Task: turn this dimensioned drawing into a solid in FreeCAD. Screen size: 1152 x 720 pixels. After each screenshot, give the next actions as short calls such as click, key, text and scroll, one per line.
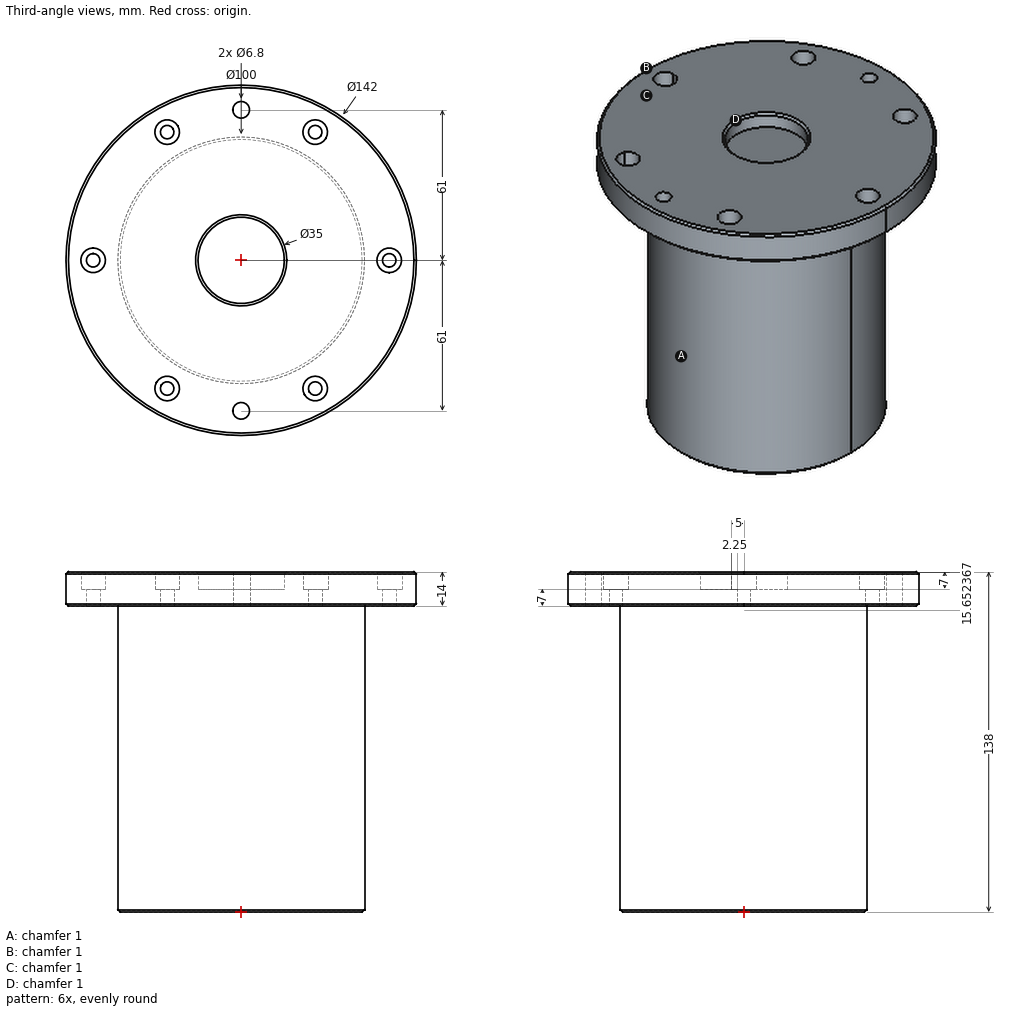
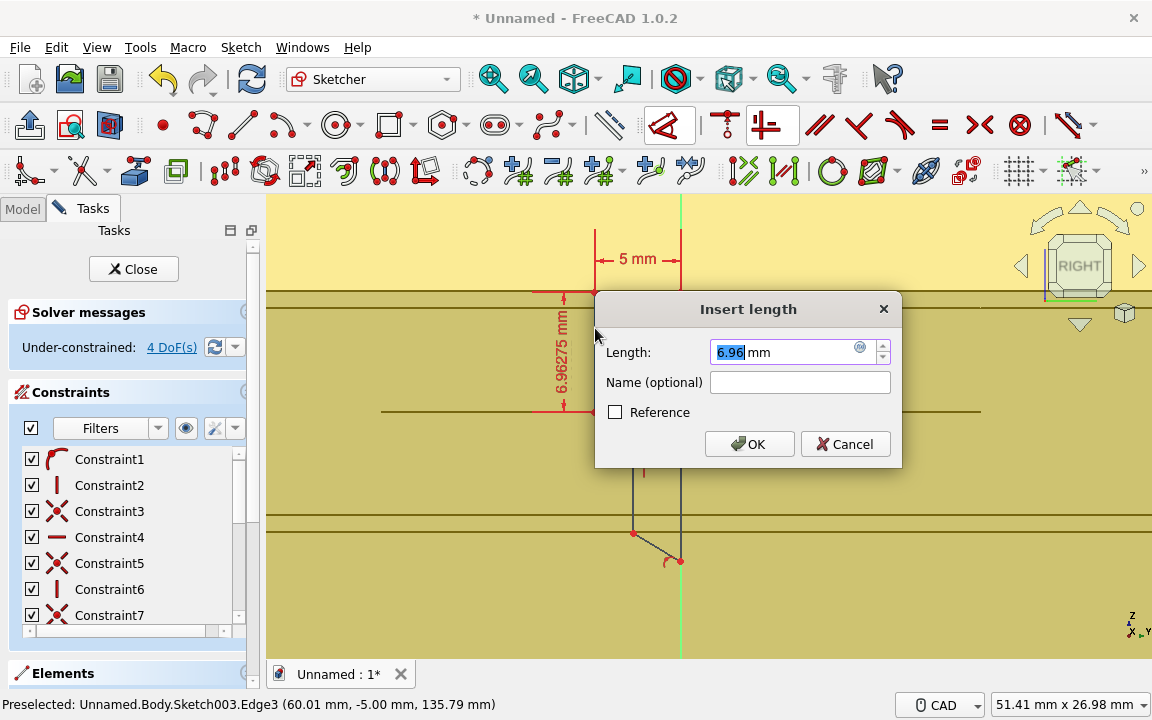
text(7)
key(Return)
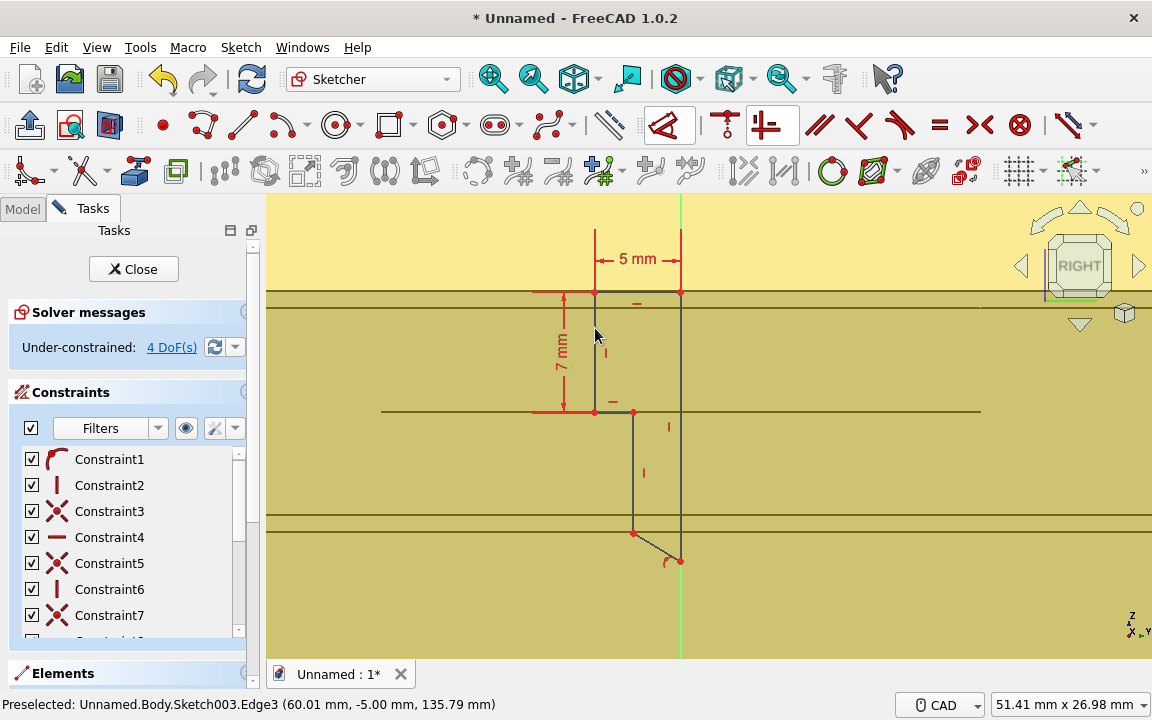
click(633, 449)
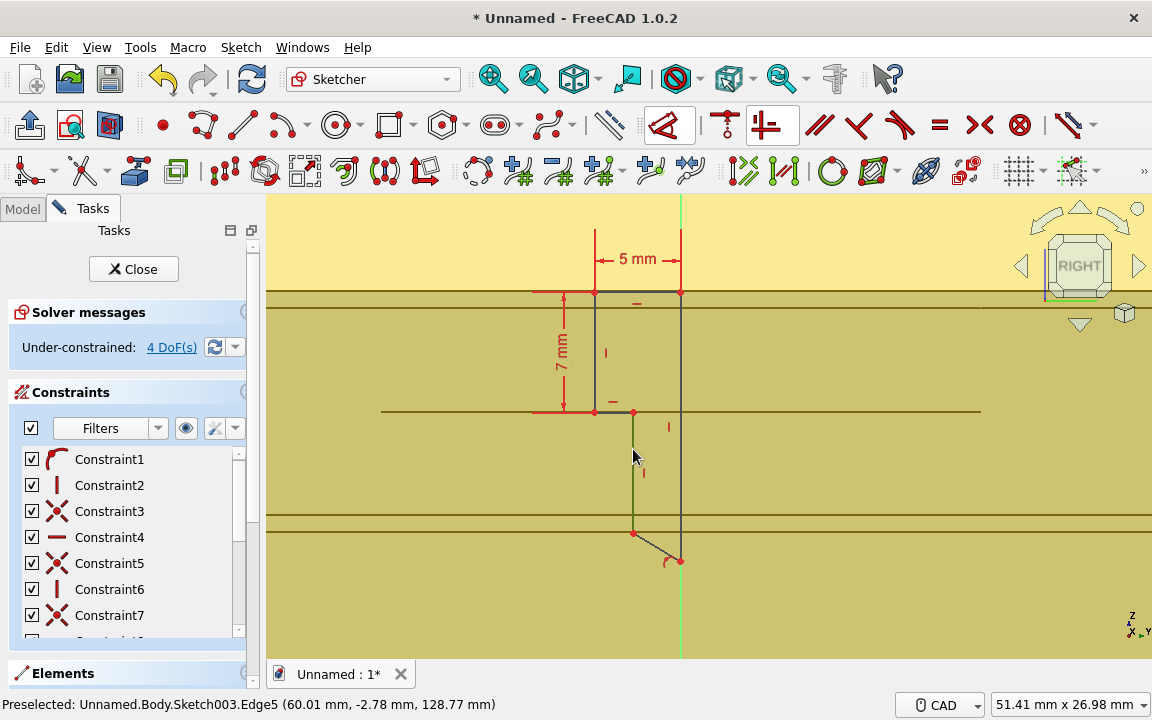
click(690, 126)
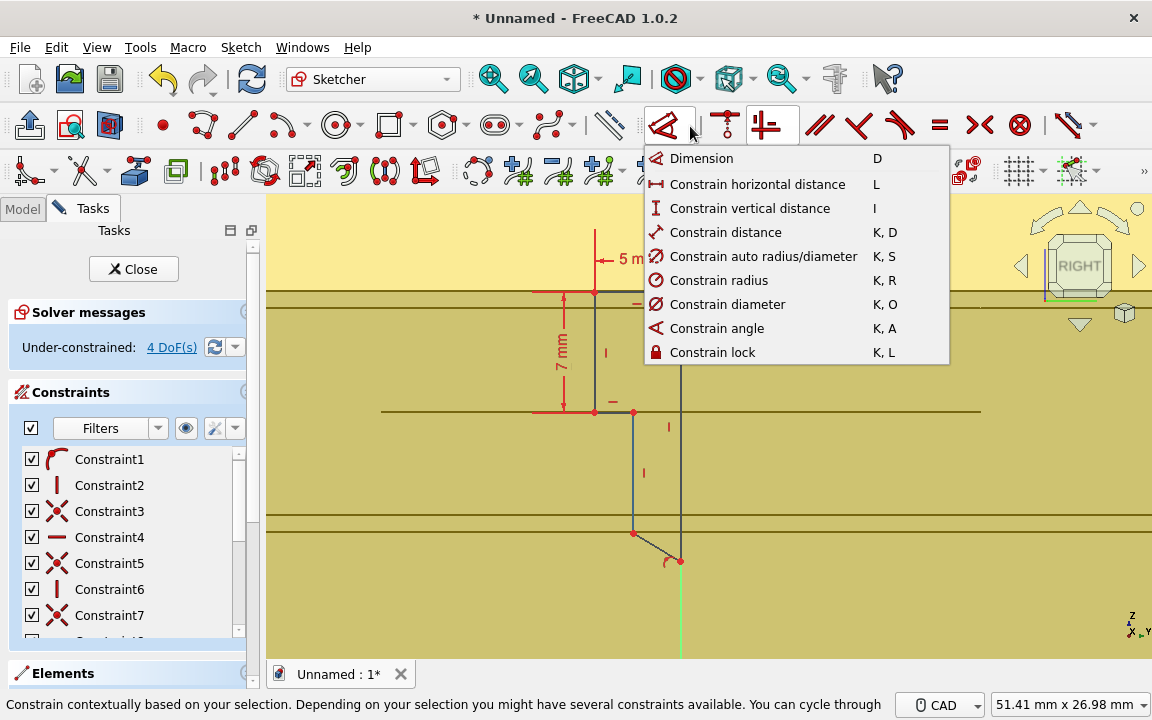
click(797, 208)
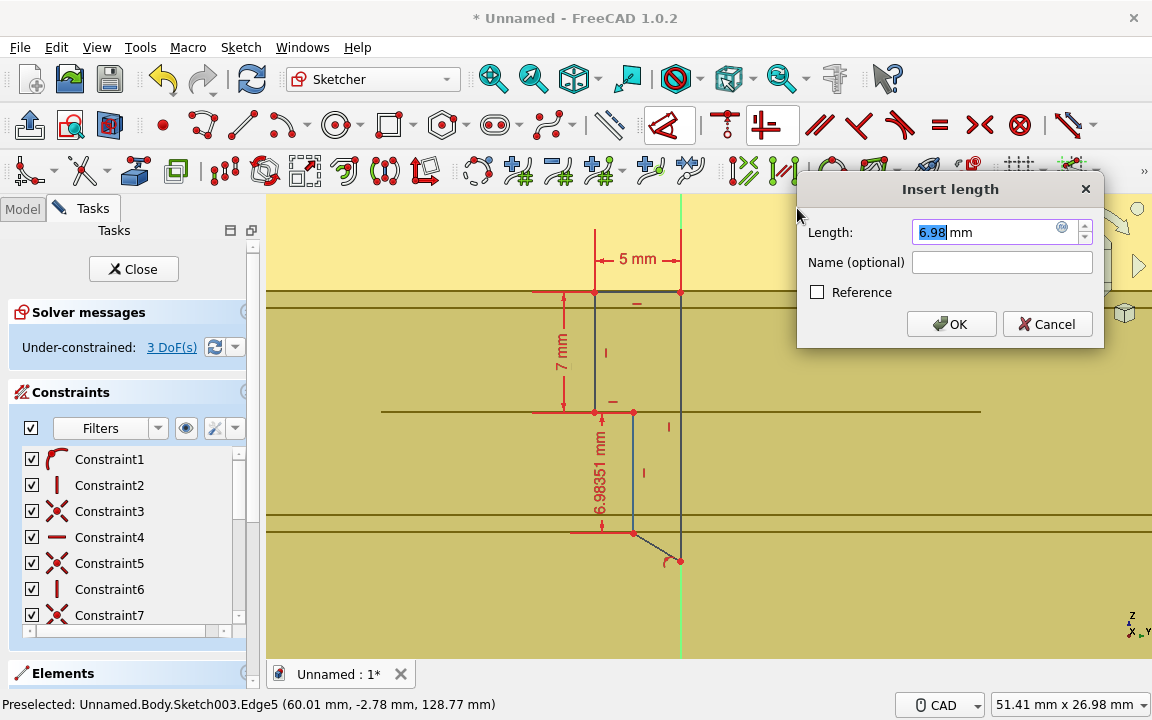
text(7)
key(Return)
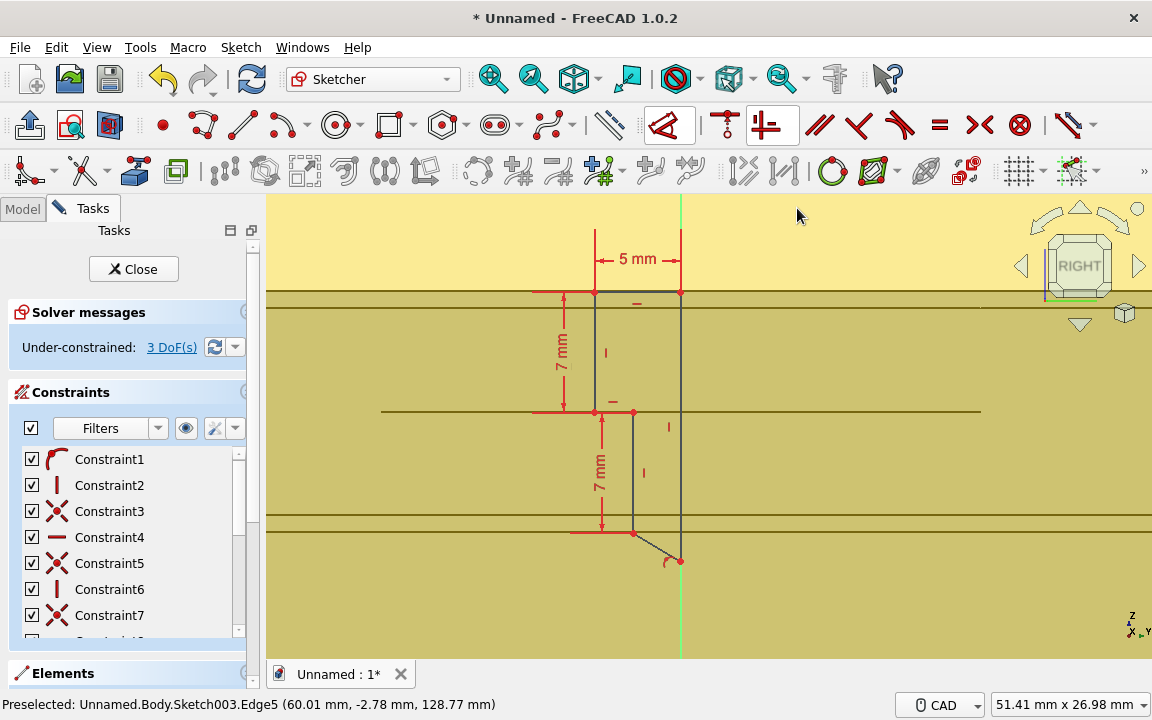
click(606, 413)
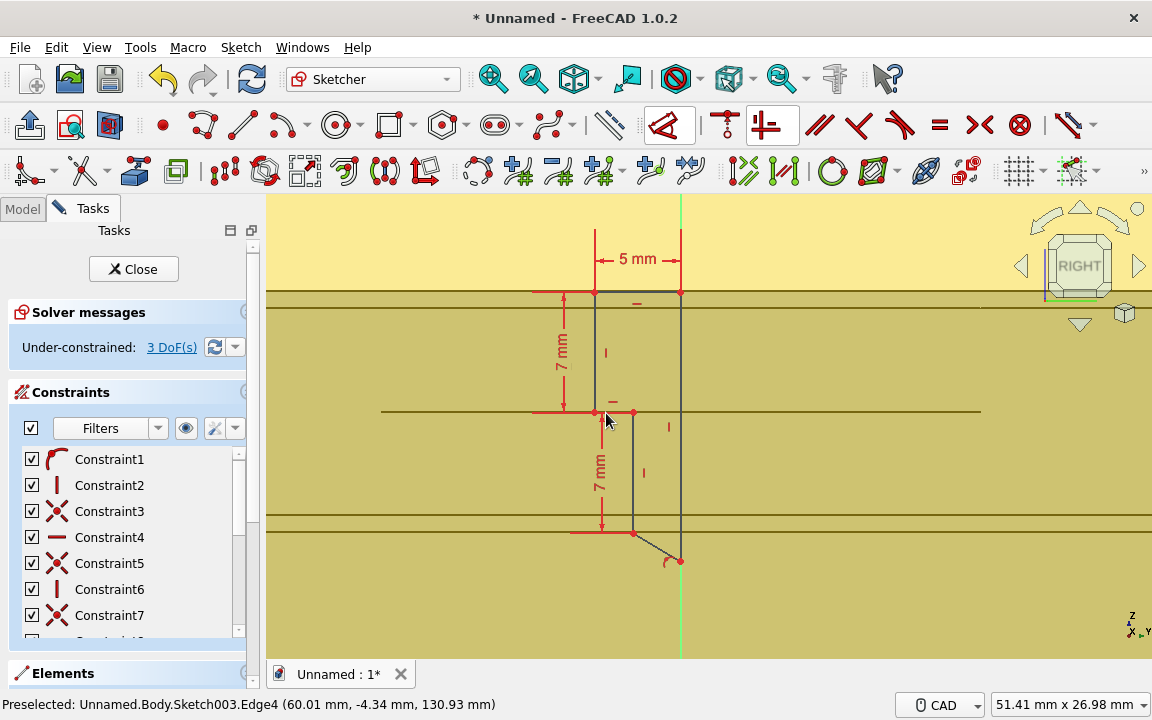
key(l)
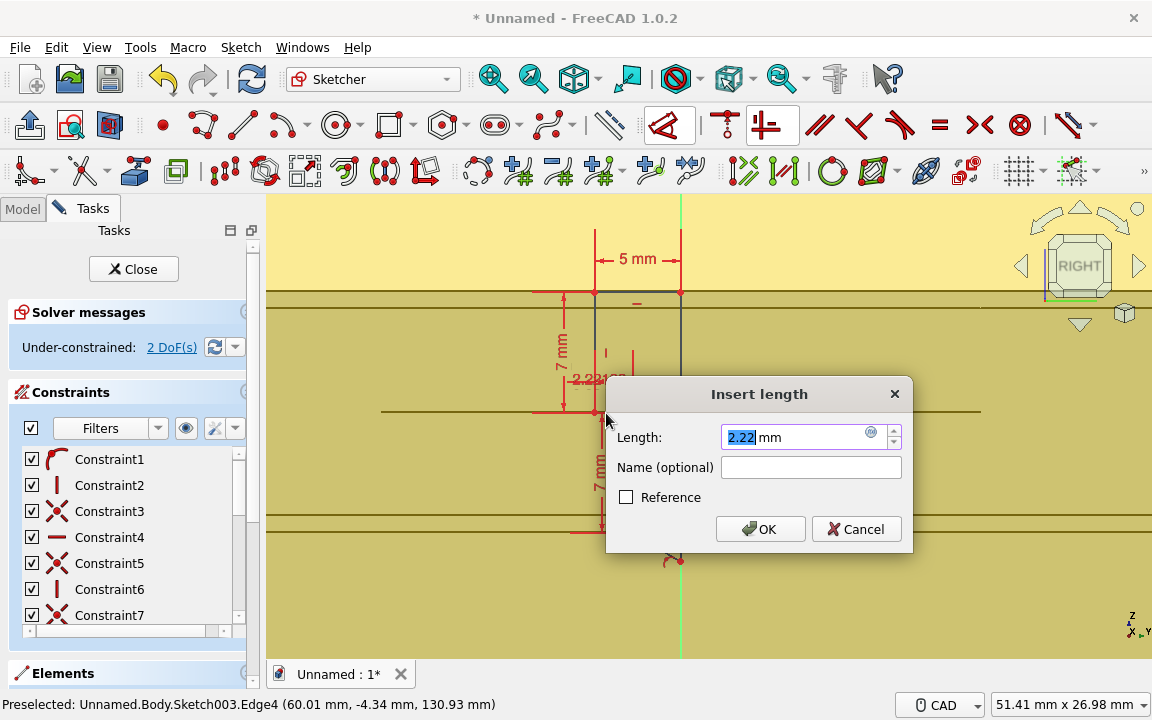
text(2.25)
key(Return)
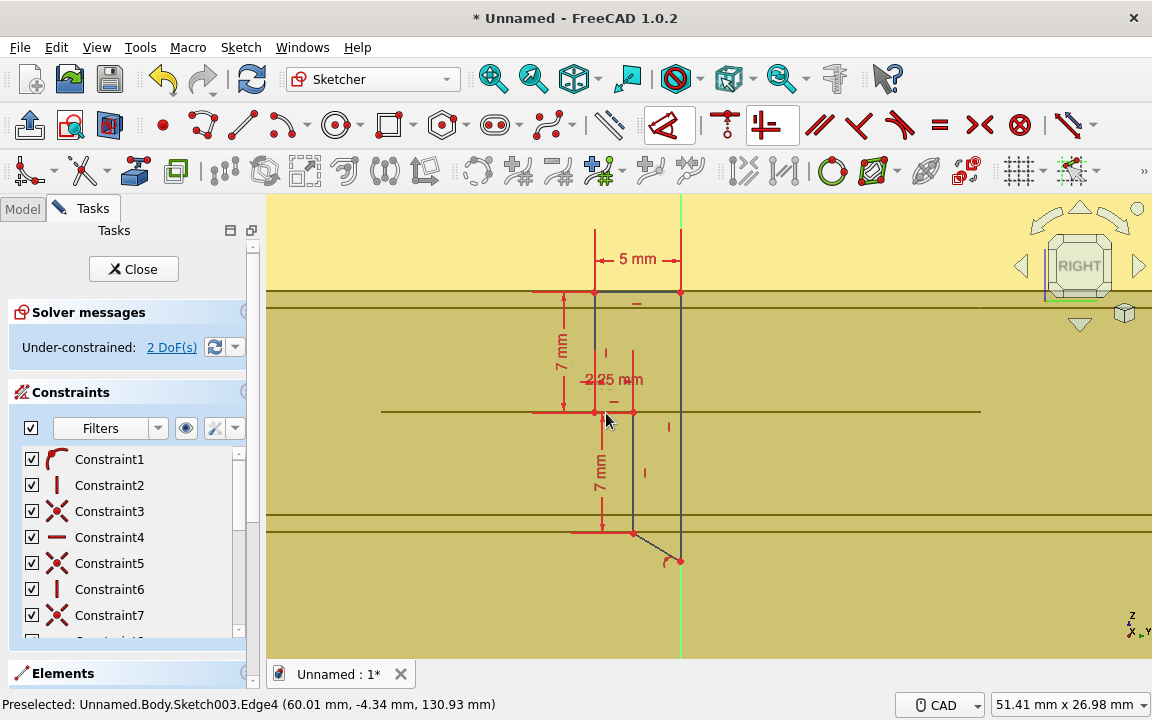
click(681, 292)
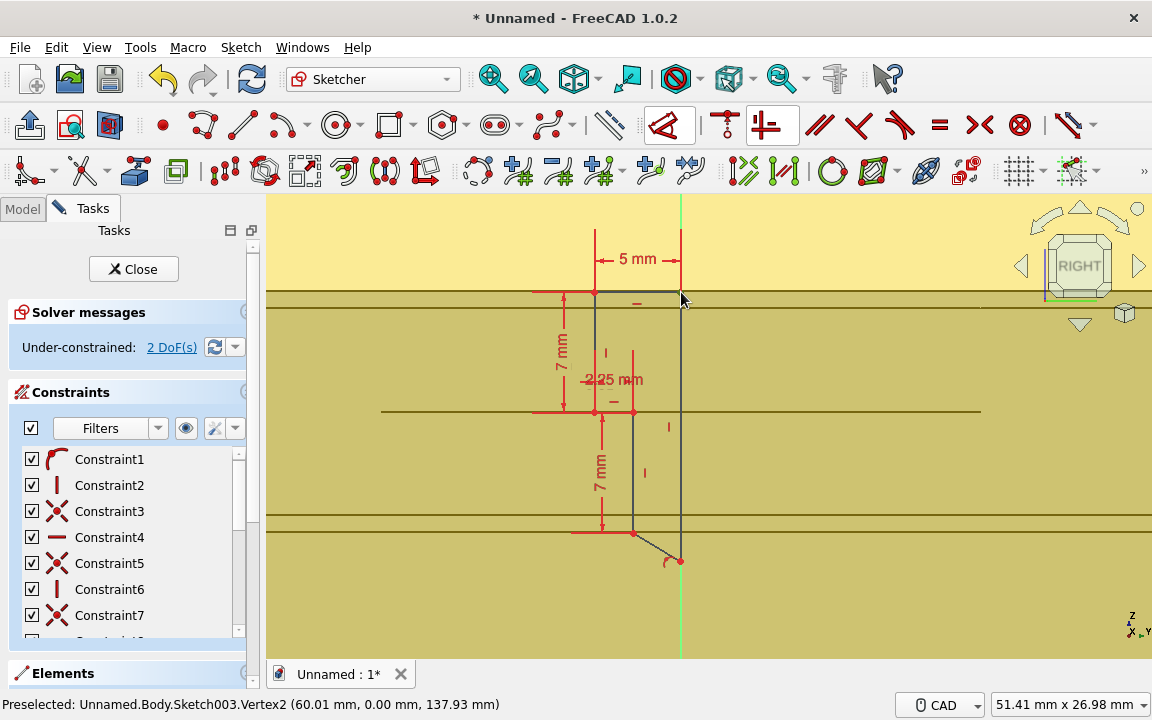
key(i)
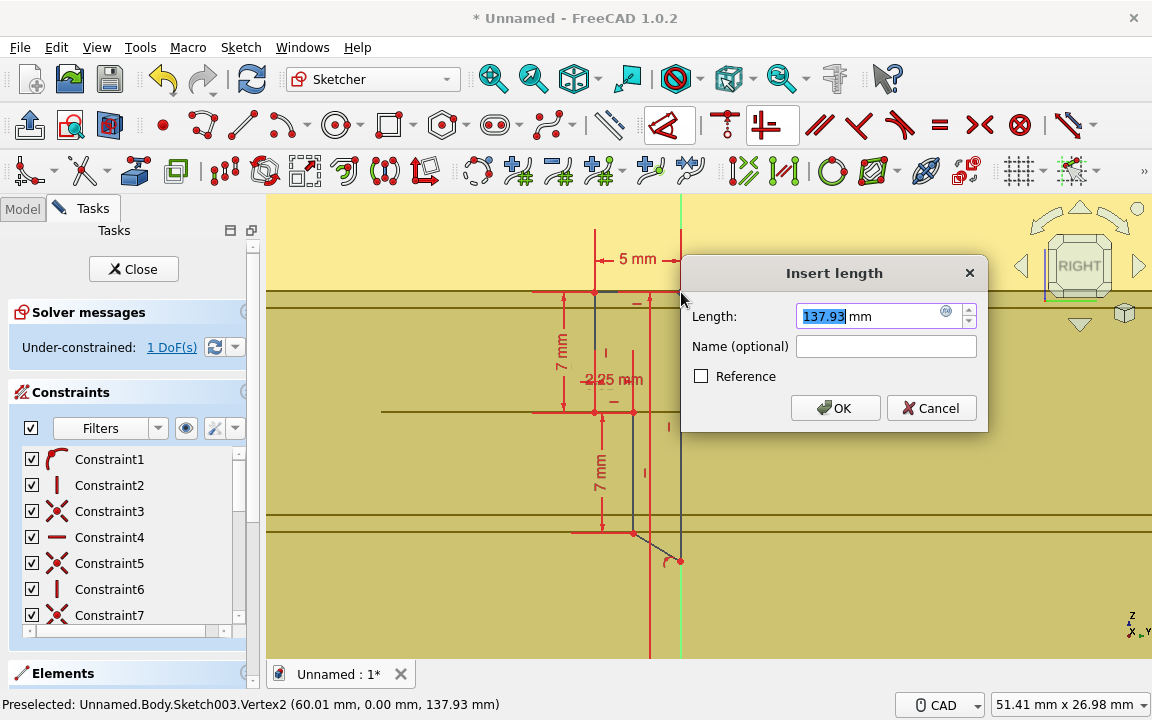
text(138)
key(Return)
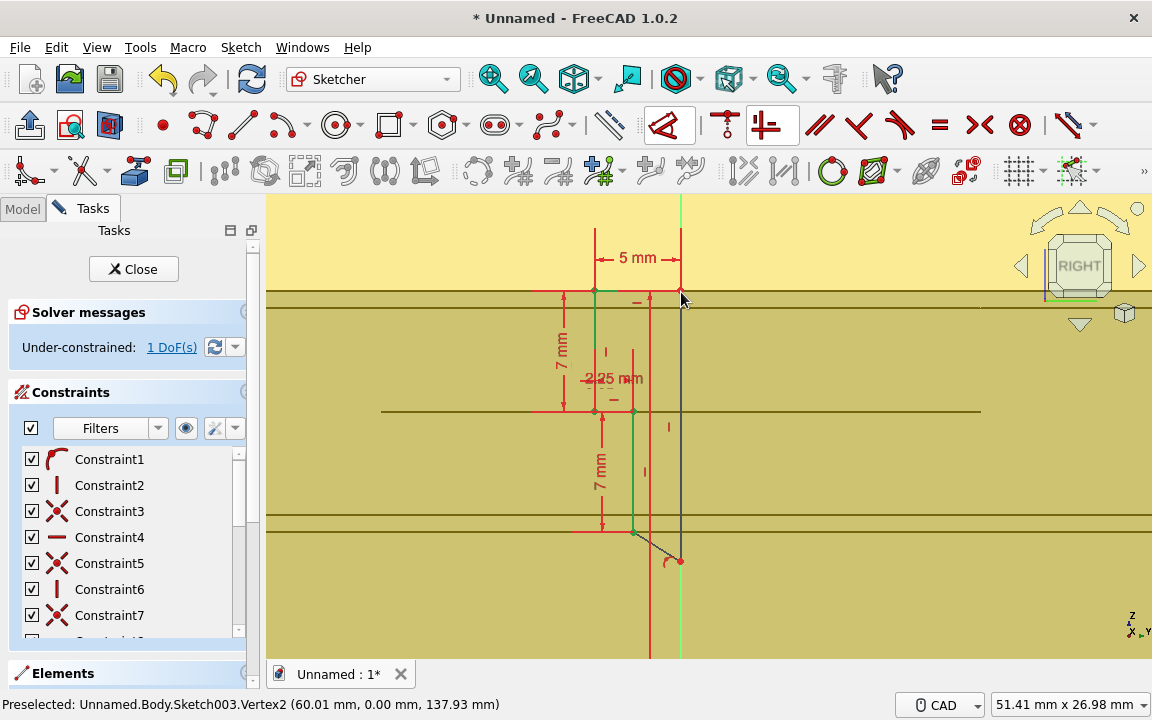
click(681, 481)